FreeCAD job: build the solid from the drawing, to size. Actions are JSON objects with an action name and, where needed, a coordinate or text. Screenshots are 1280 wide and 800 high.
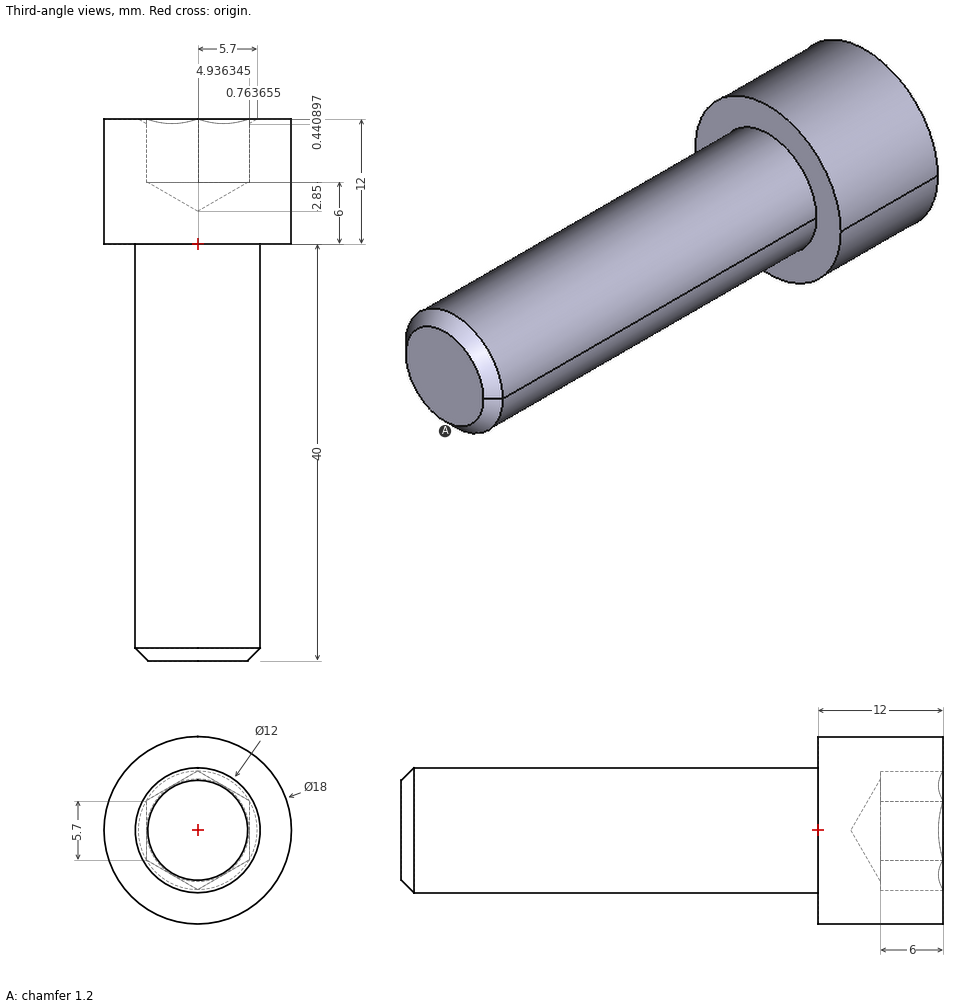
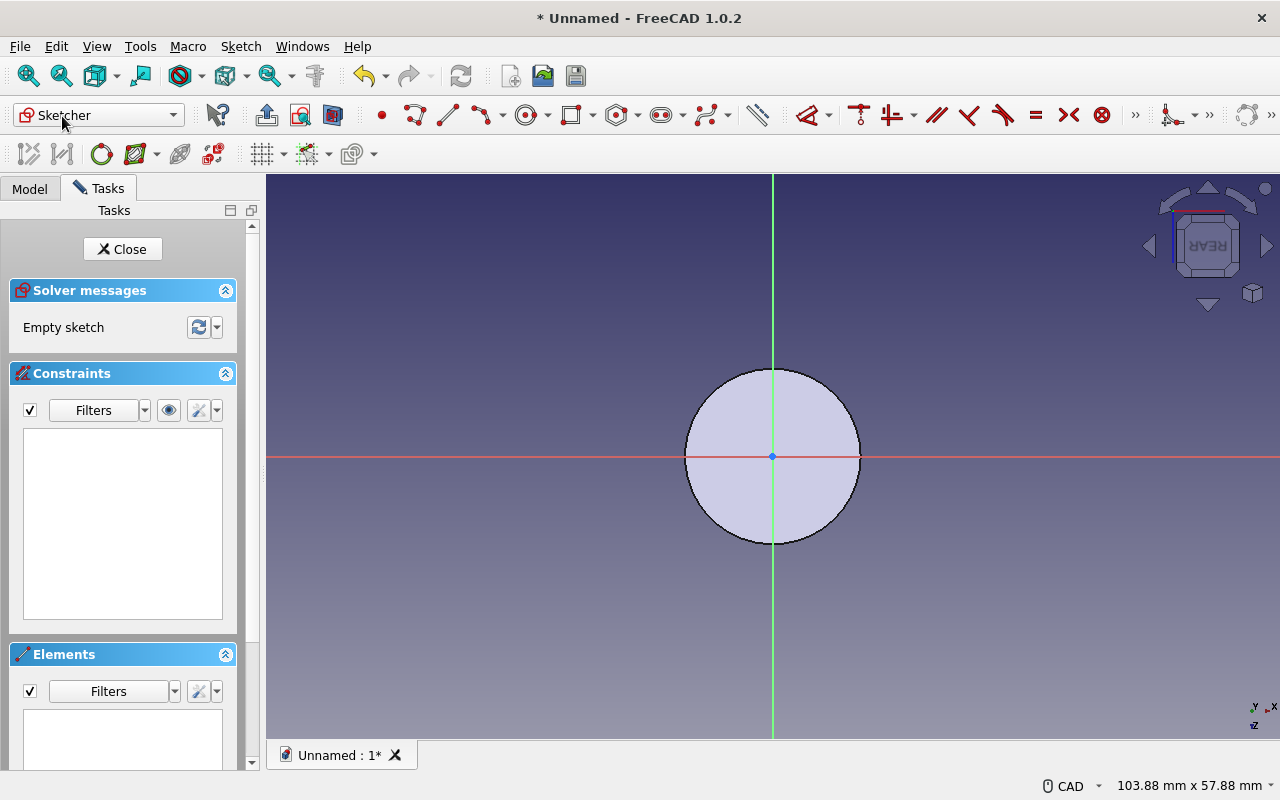
{"action": "scroll", "coordinate": [802, 456], "scroll_direction": "up", "scroll_amount": 6}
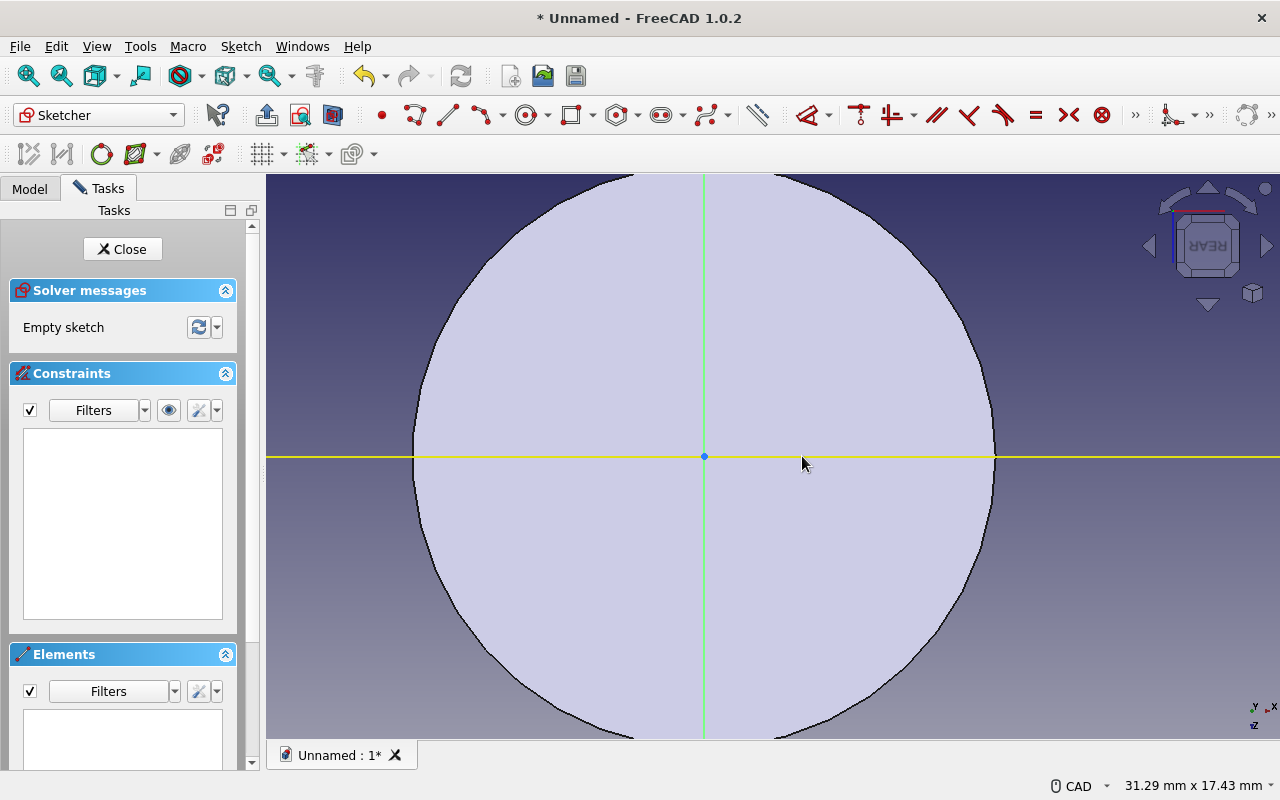
{"action": "left_click", "coordinate": [616, 116]}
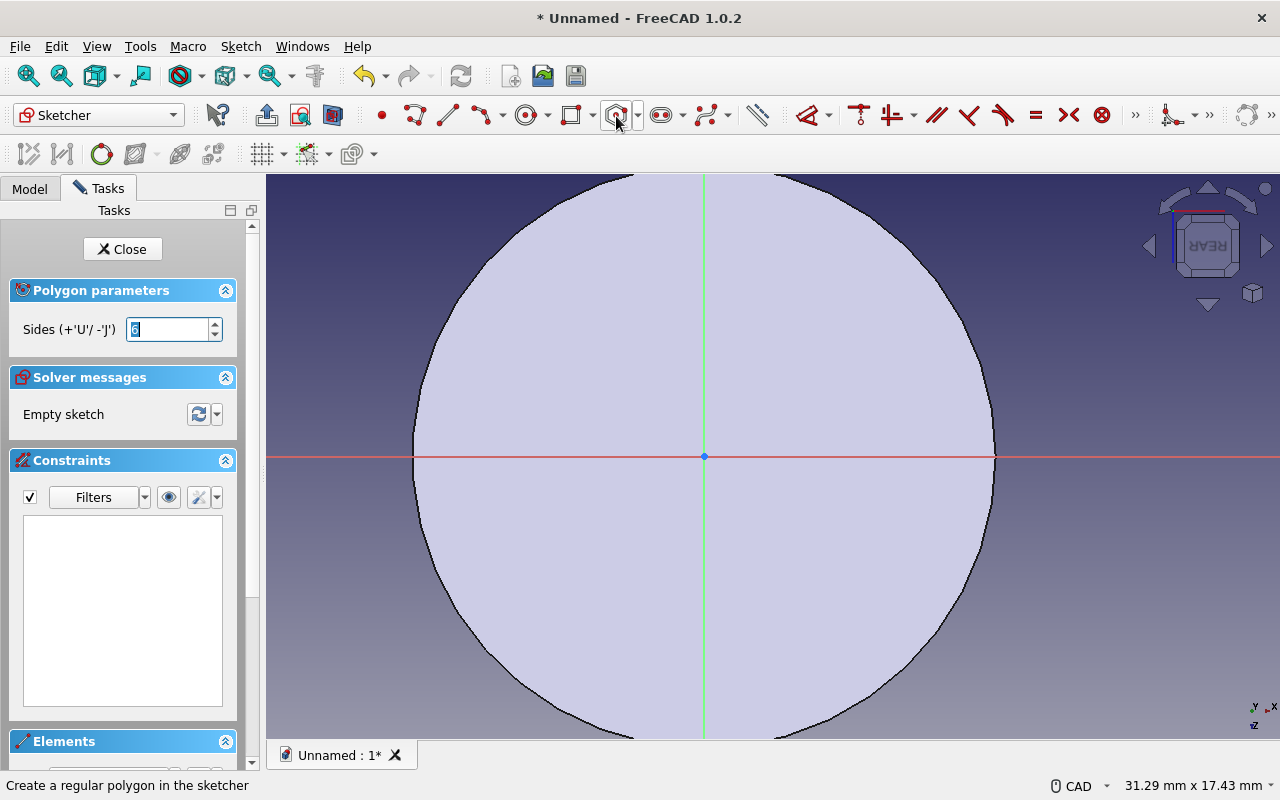
{"action": "left_click", "coordinate": [704, 456]}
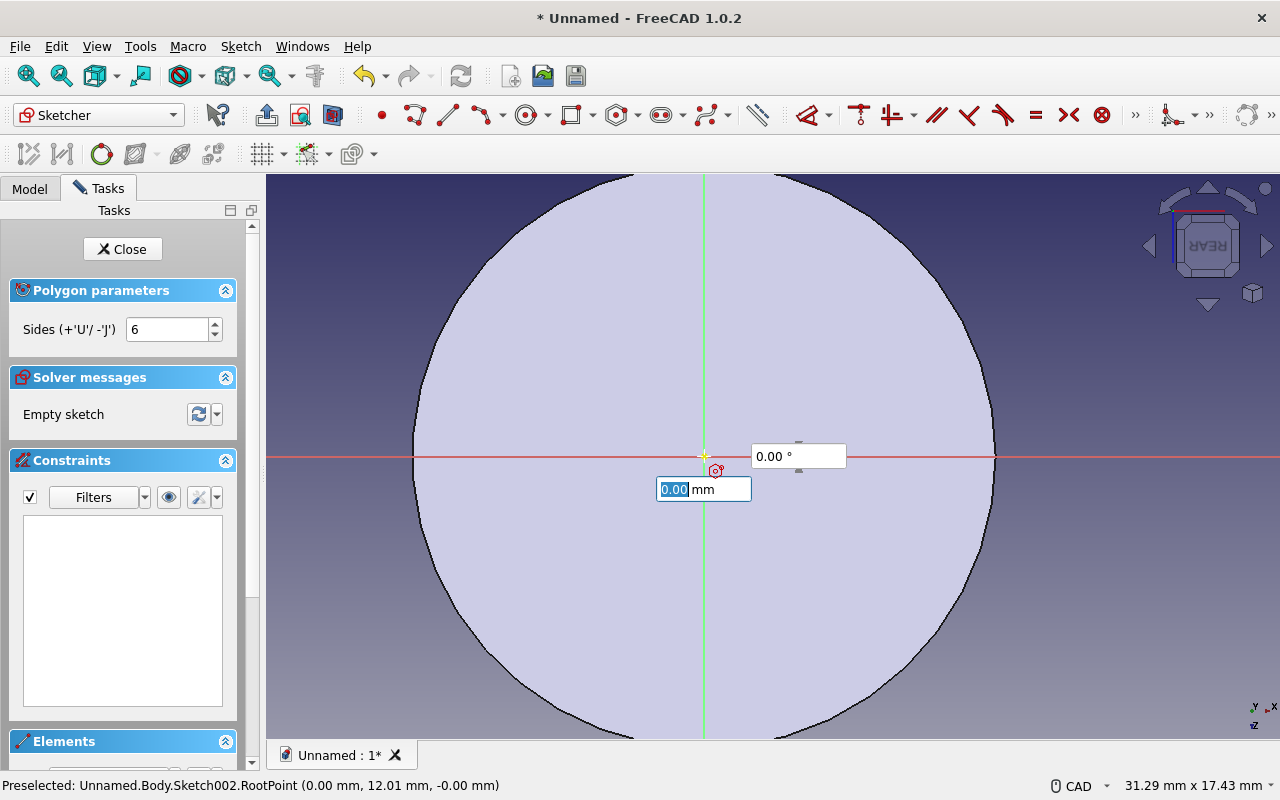
{"action": "left_click", "coordinate": [704, 272]}
{"action": "key", "text": "Escape"}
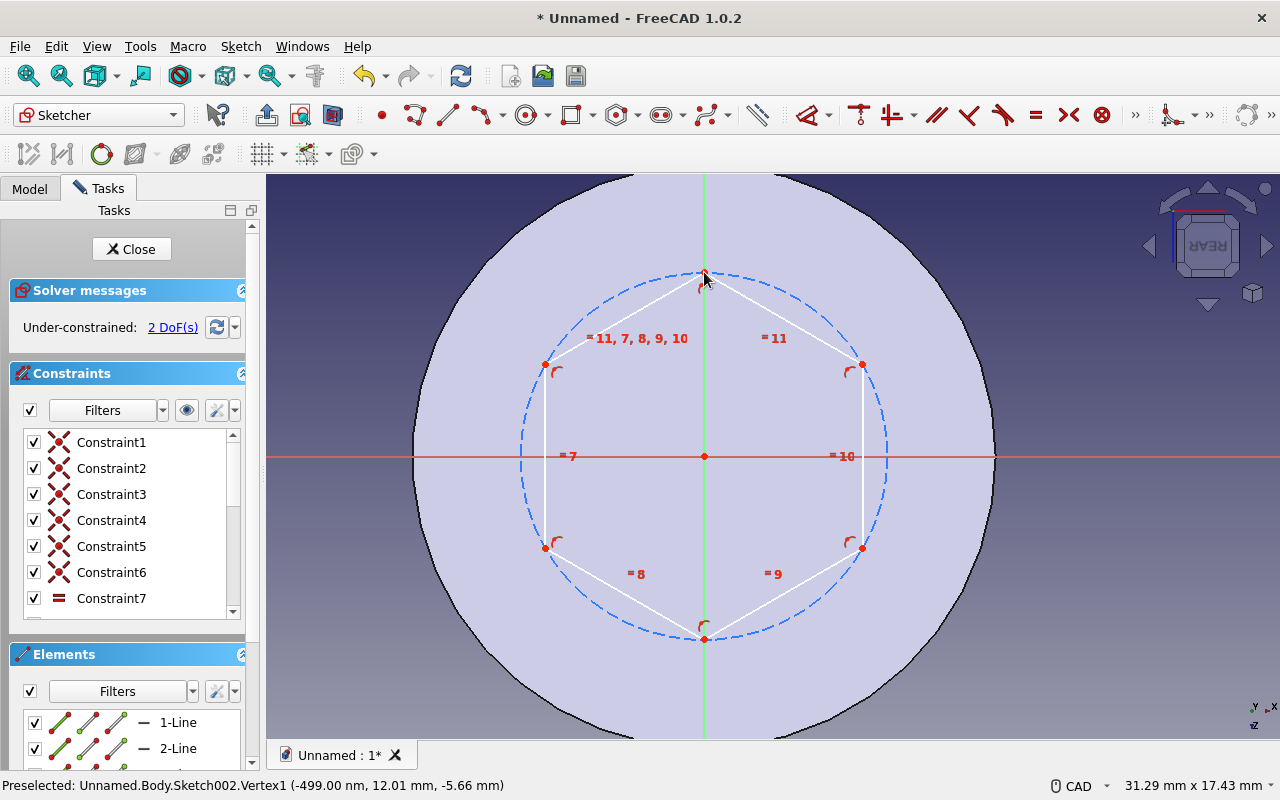
{"action": "left_click", "coordinate": [545, 420]}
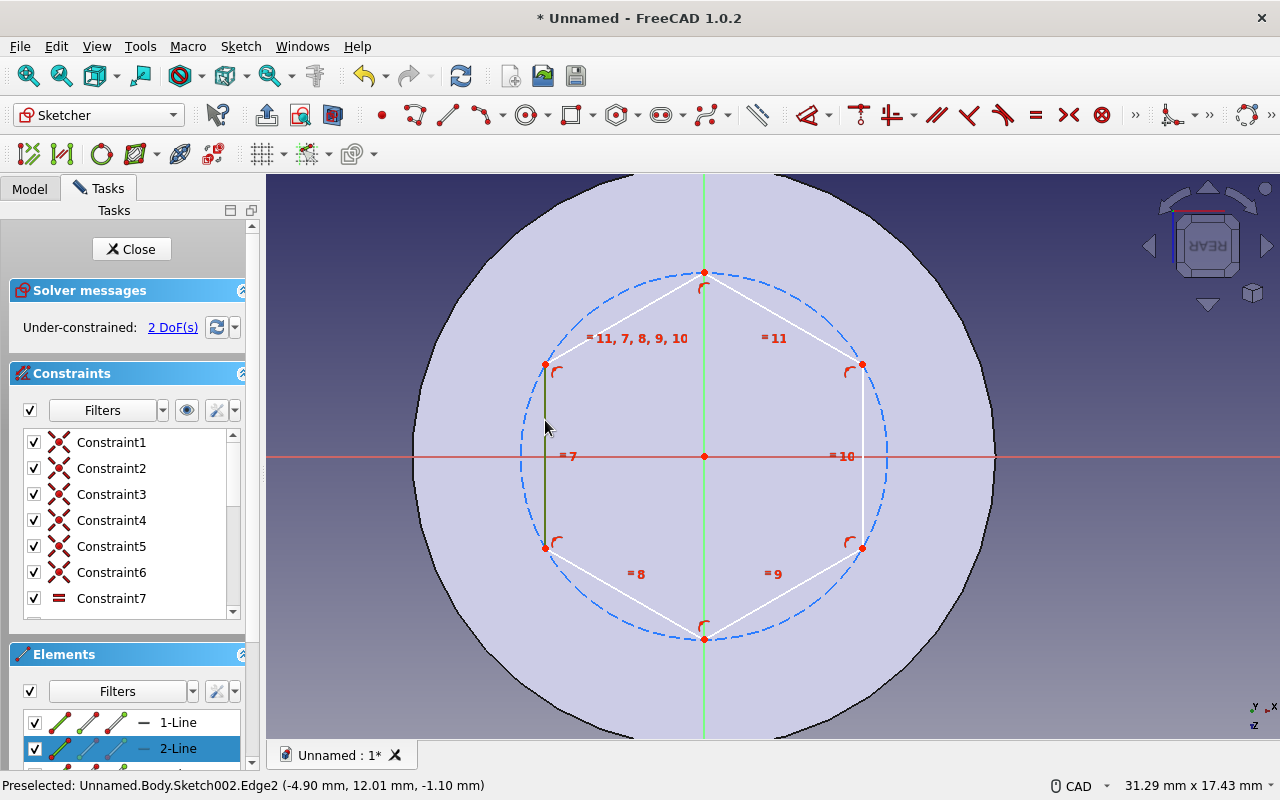
{"action": "key", "text": "v"}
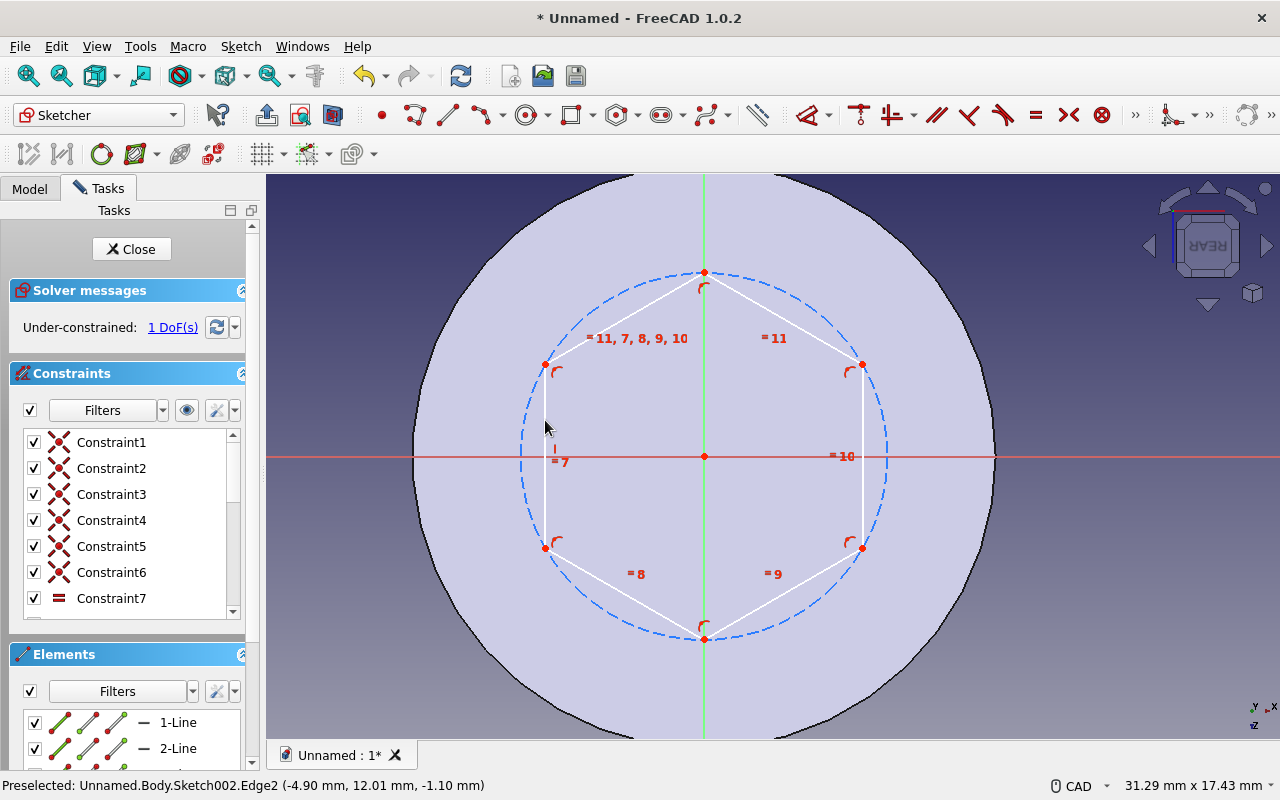
{"action": "left_click", "coordinate": [806, 116]}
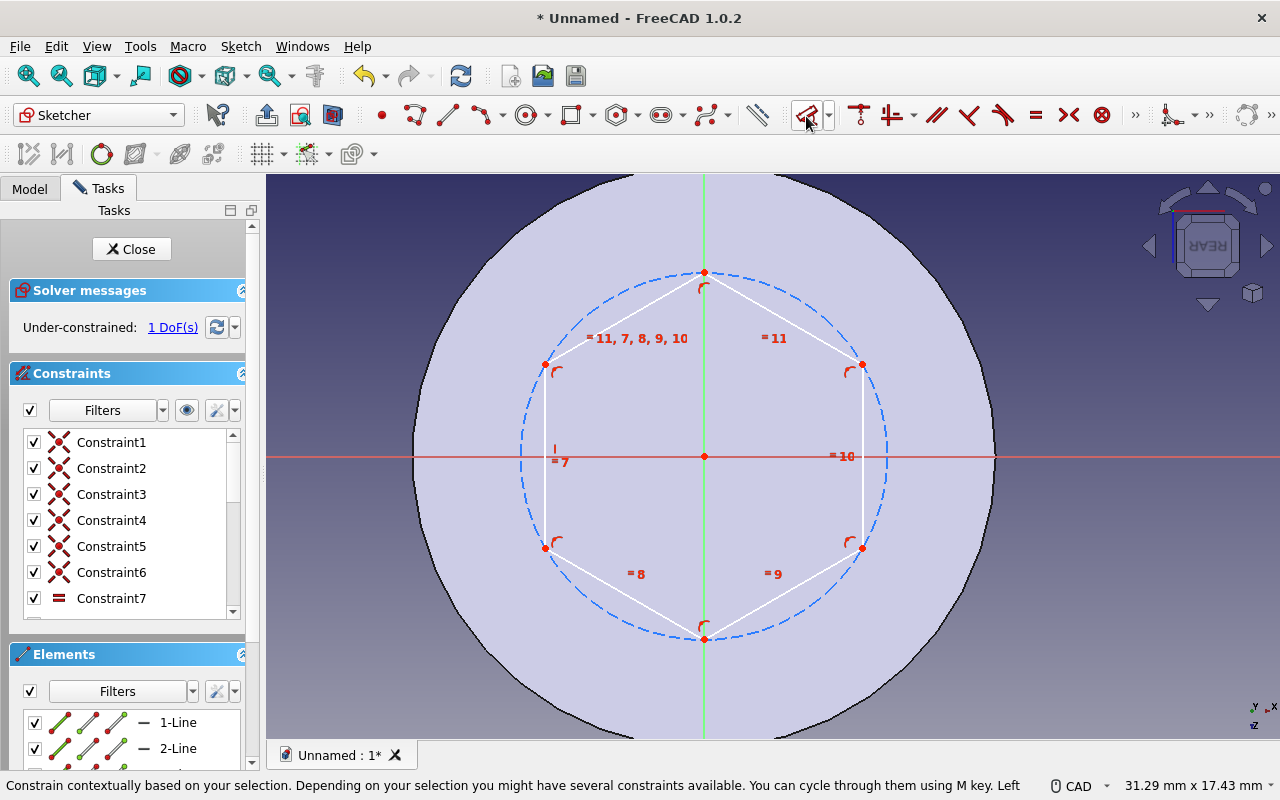
{"action": "left_click", "coordinate": [545, 420]}
{"action": "left_click", "coordinate": [511, 414]}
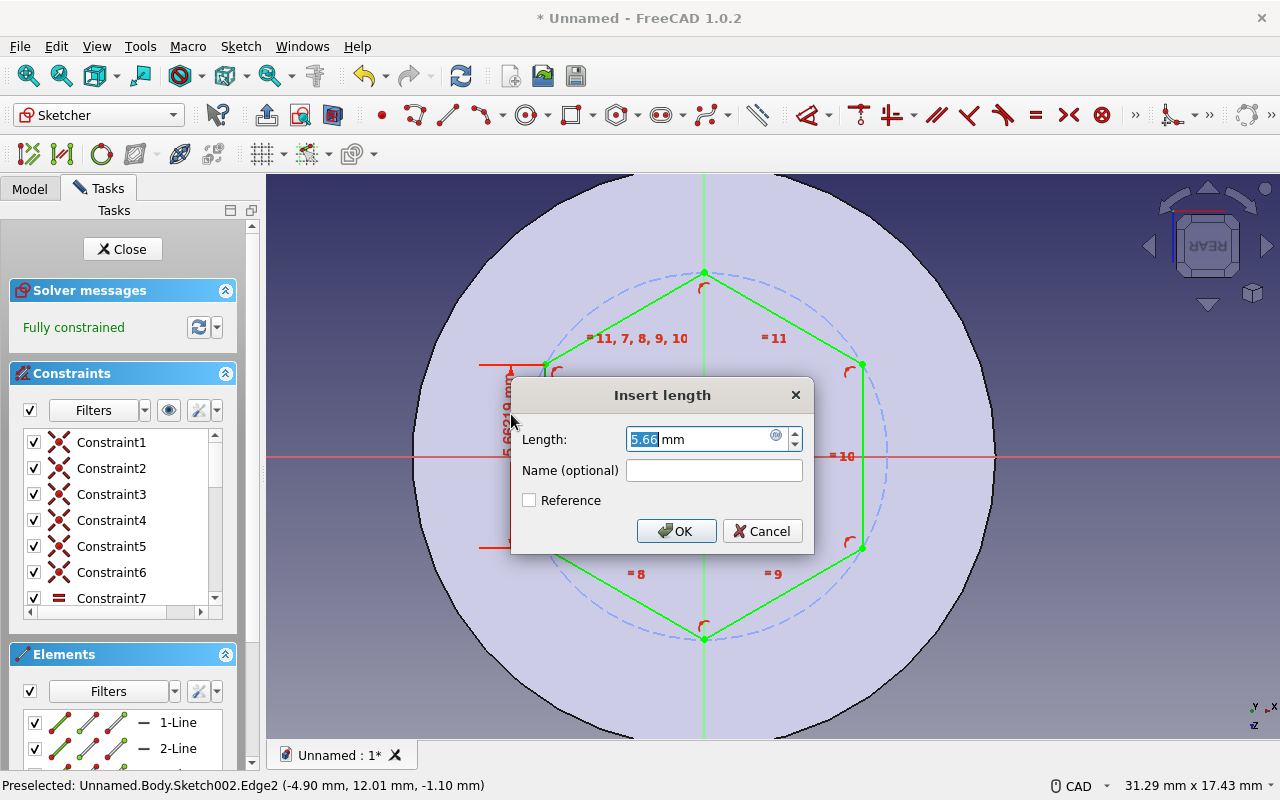
{"action": "type", "text": "5.7"}
{"action": "key", "text": "Return"}
{"action": "key", "text": "Escape"}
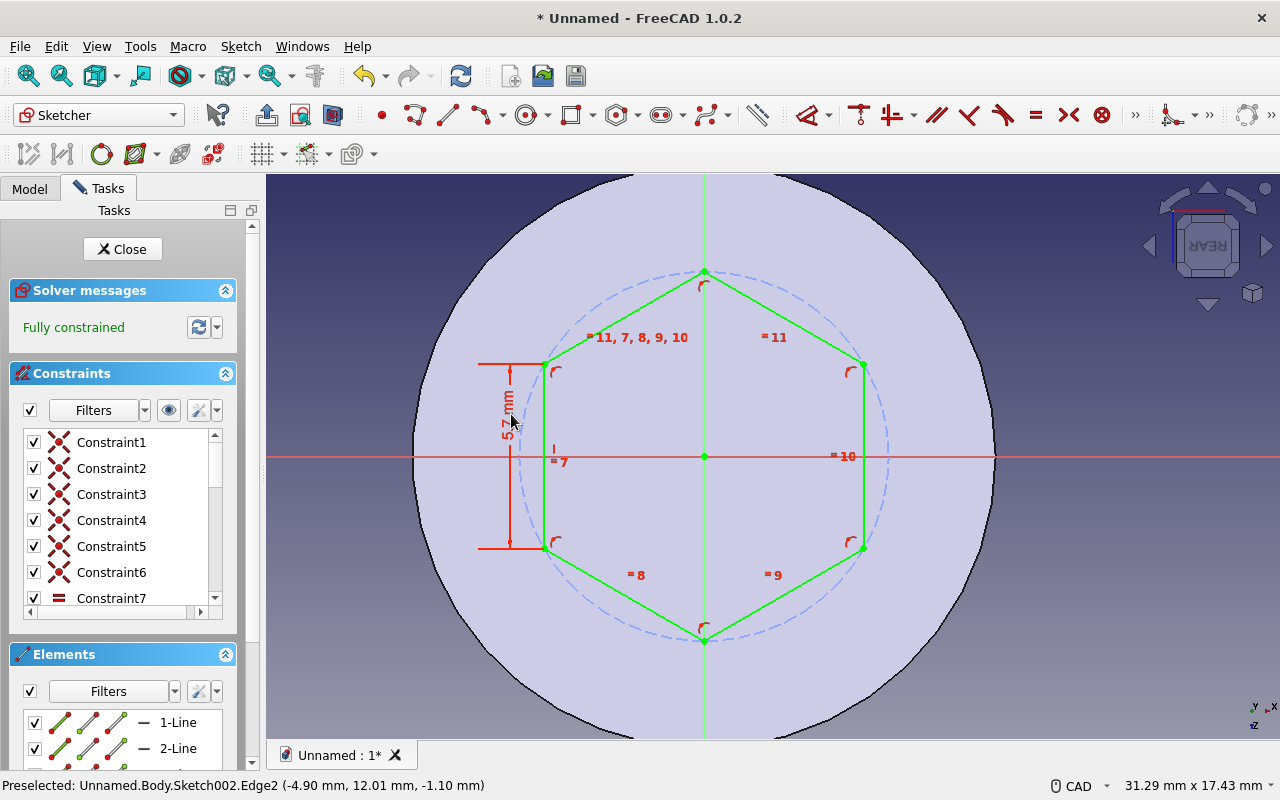
{"action": "left_click", "coordinate": [123, 249]}